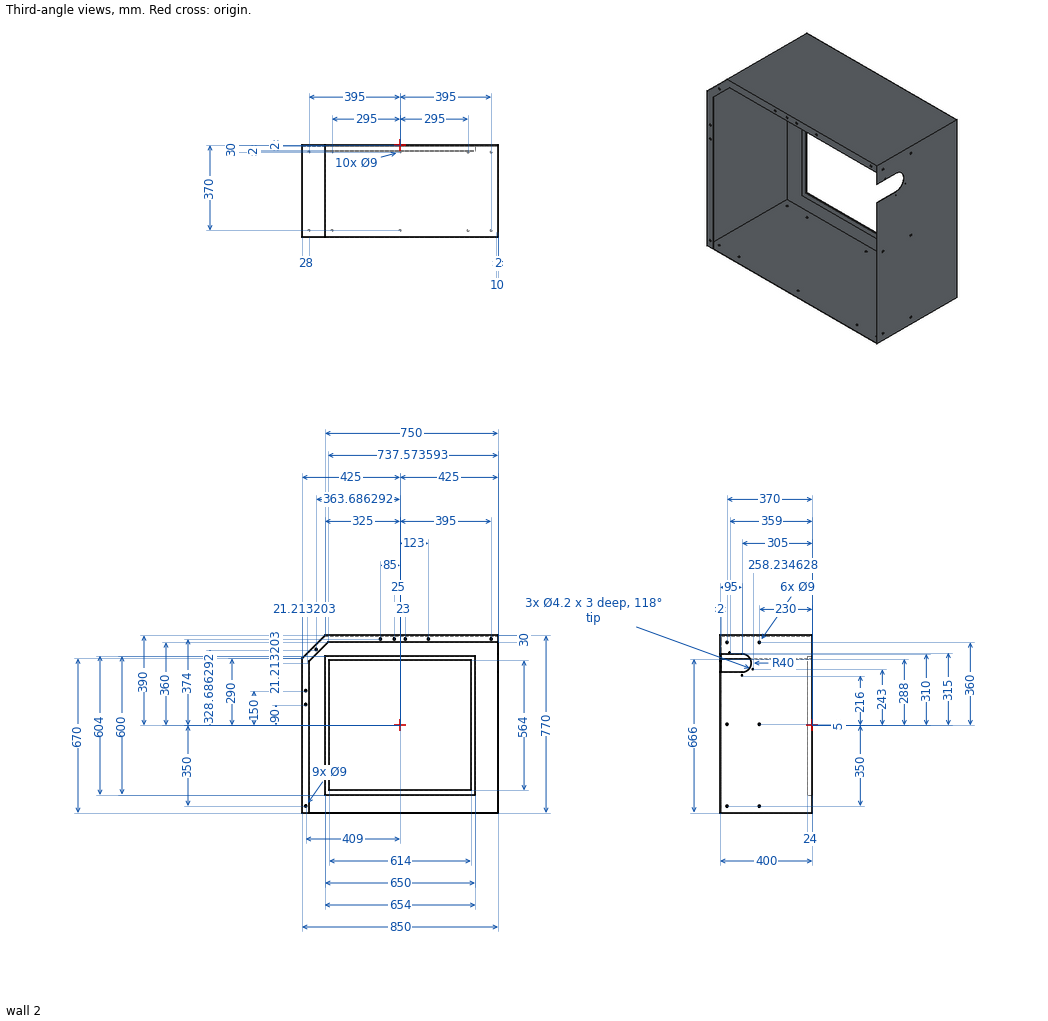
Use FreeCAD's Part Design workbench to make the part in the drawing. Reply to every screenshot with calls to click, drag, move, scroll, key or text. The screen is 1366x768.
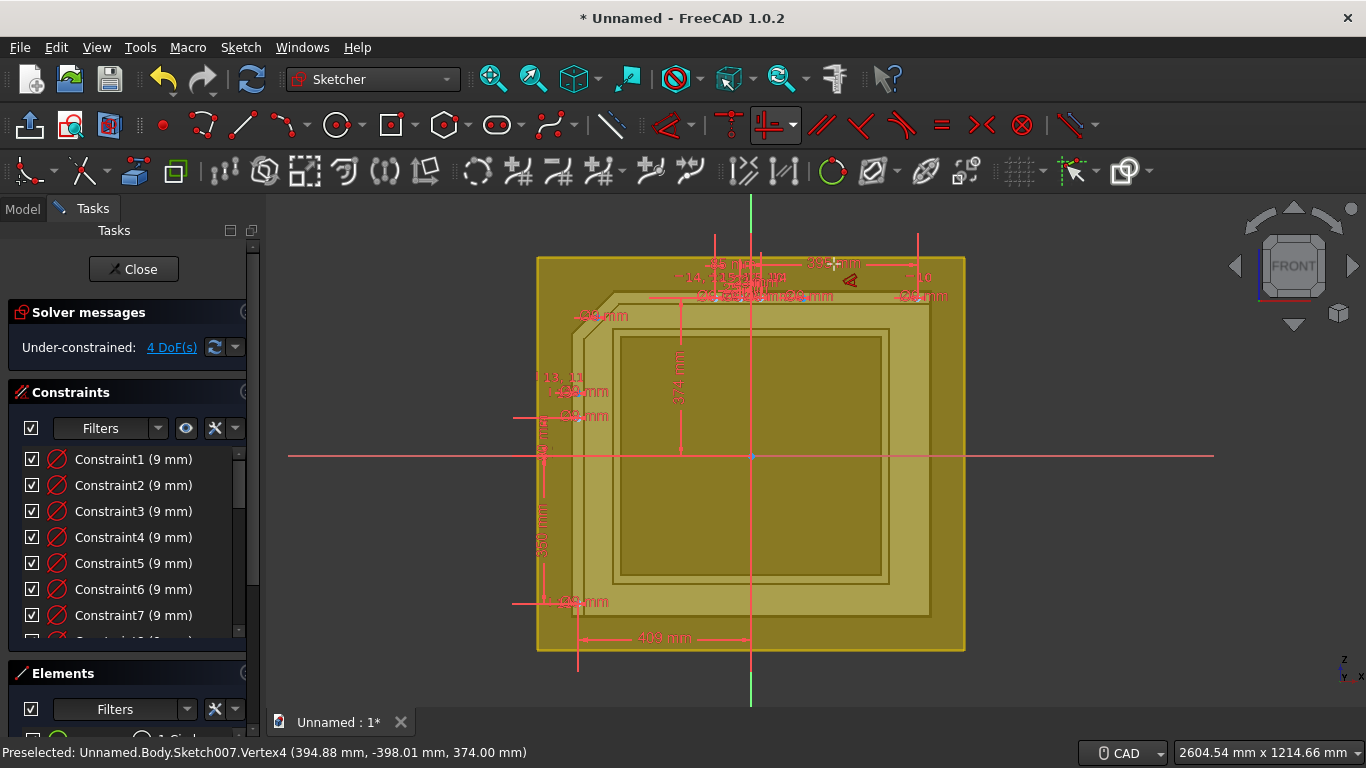
click(578, 393)
click(544, 410)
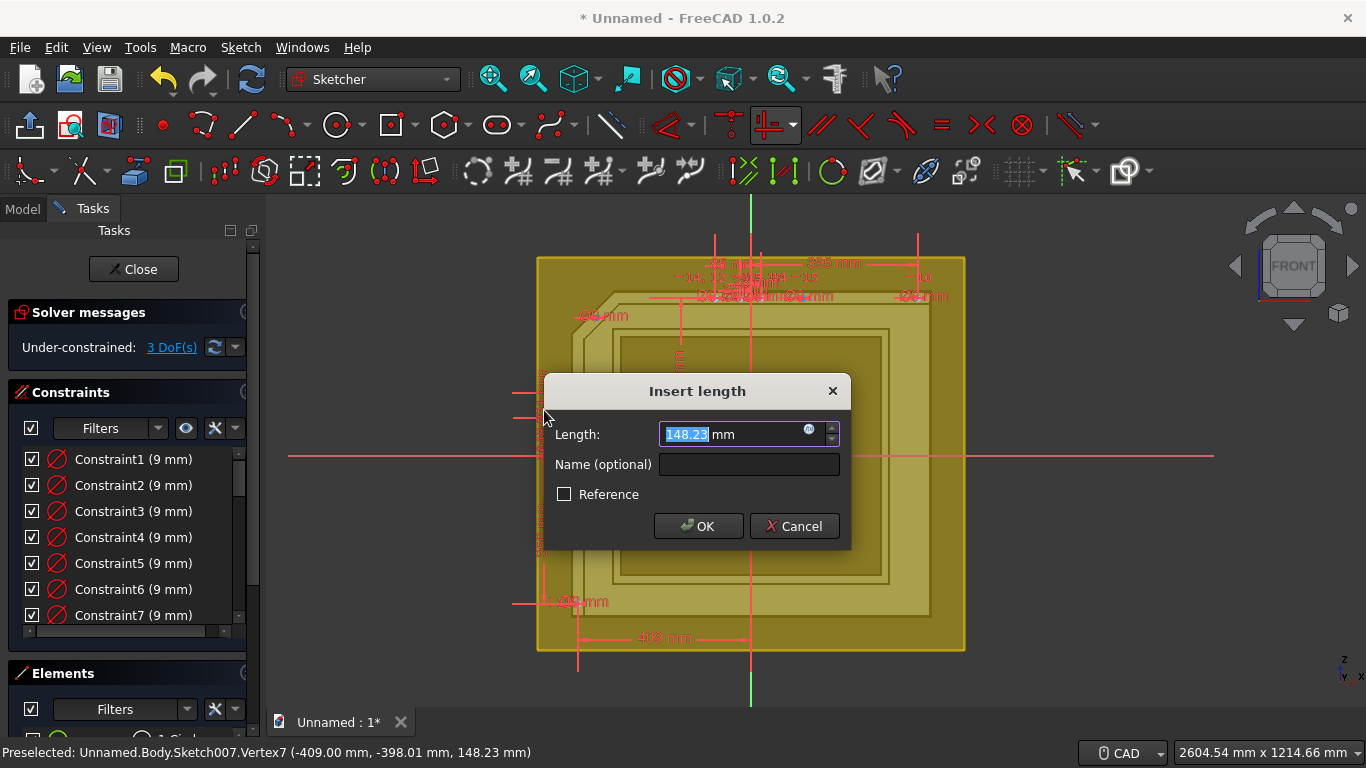
text(150)
key(Return)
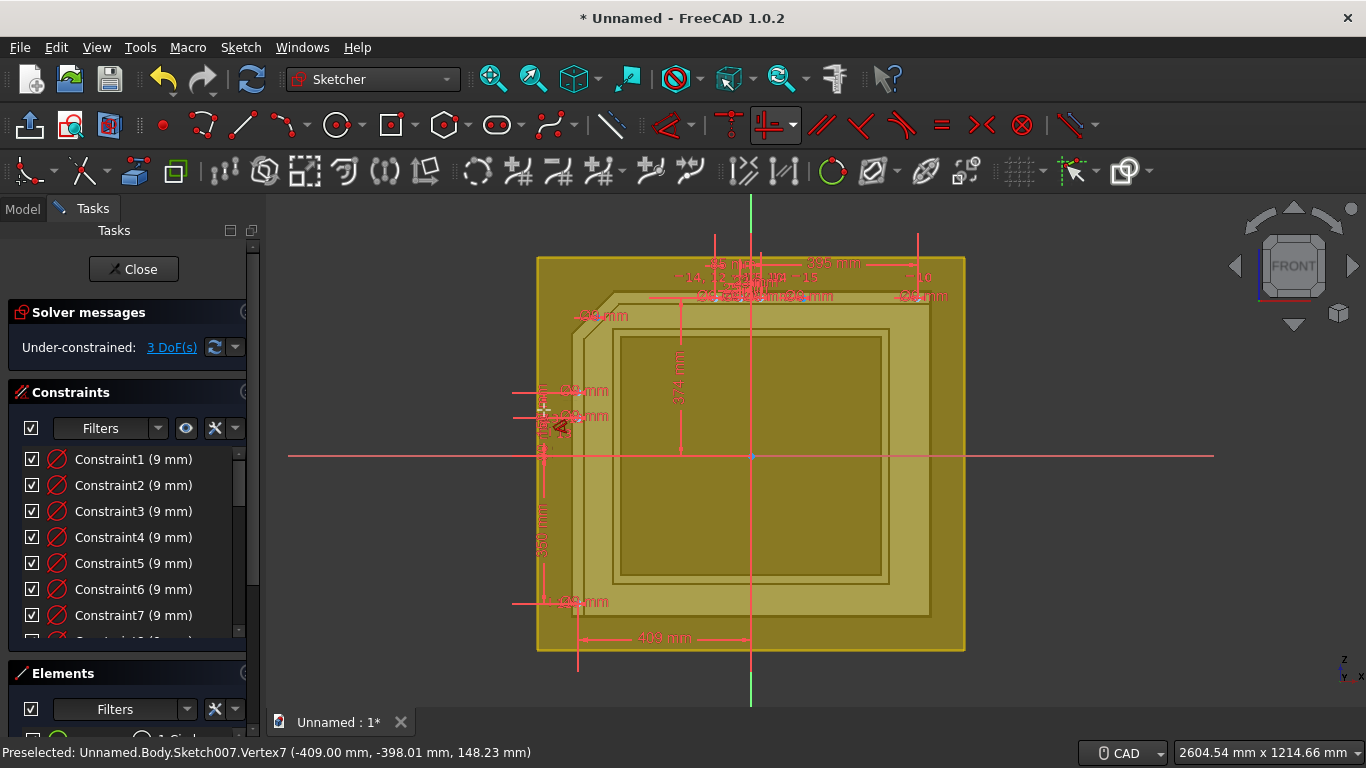
click(803, 298)
click(777, 490)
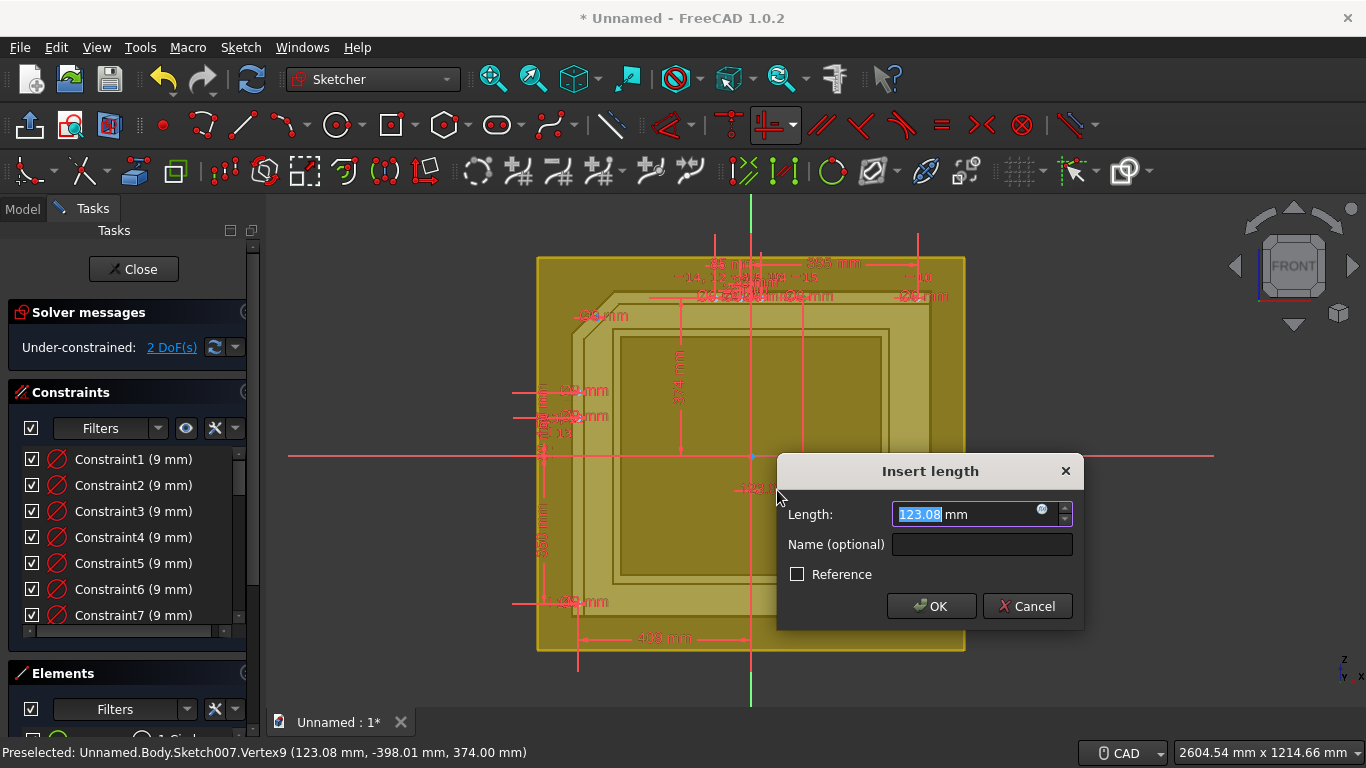
text(123)
key(Return)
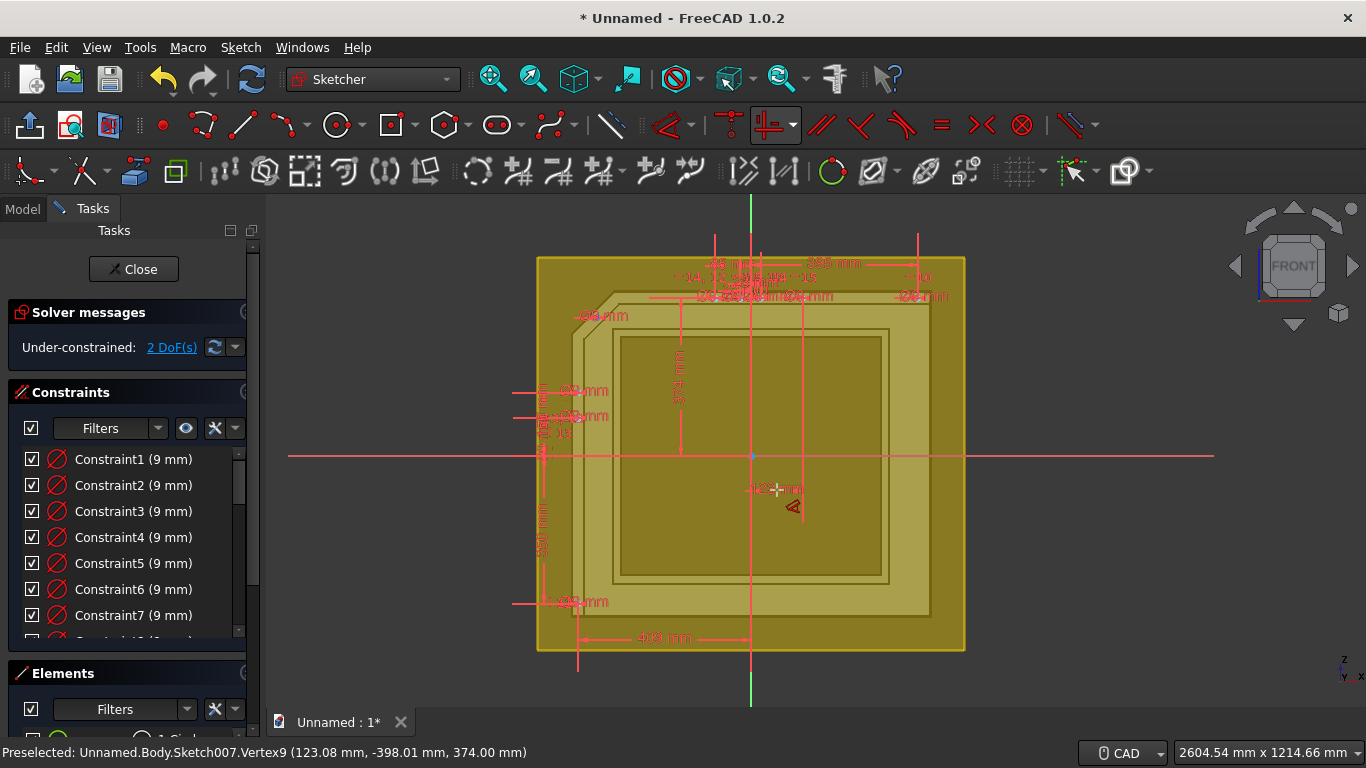
click(598, 318)
click(639, 284)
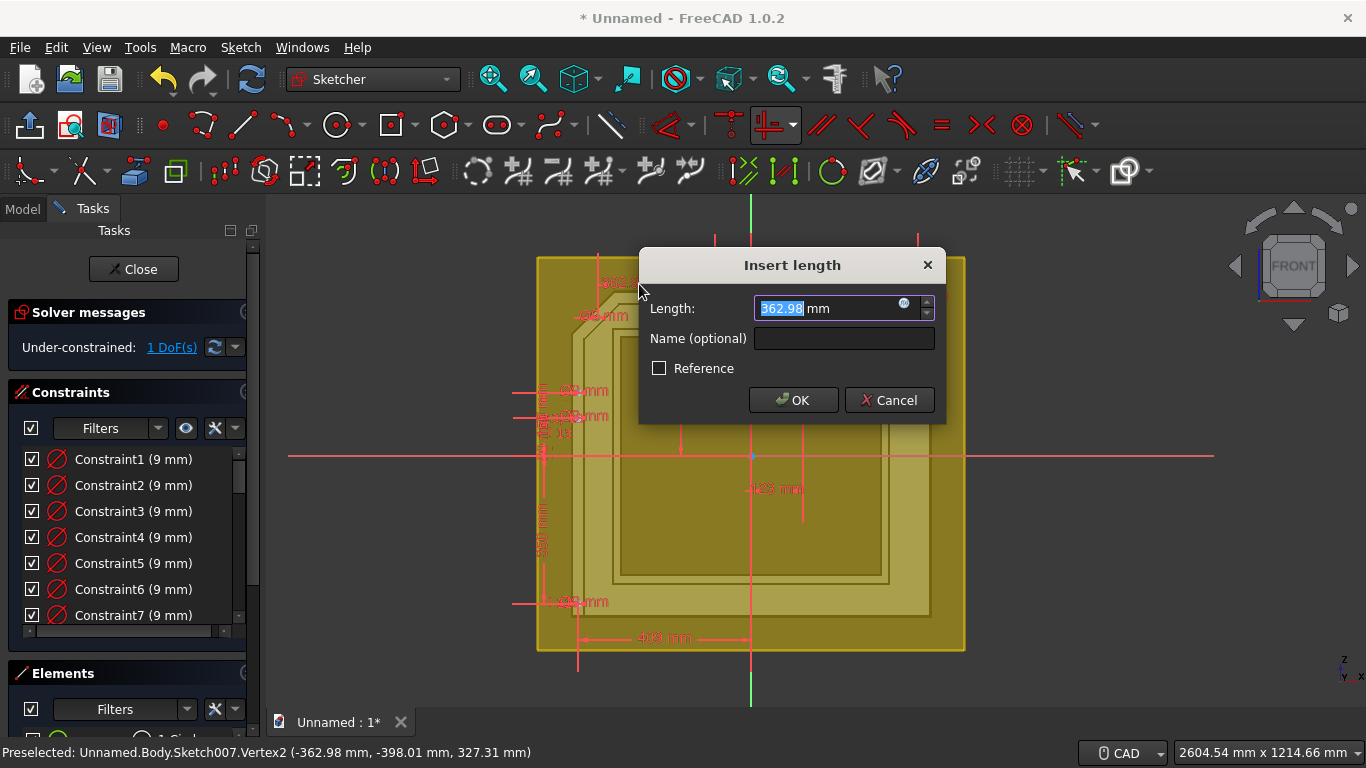
text(363.686292)
key(Return)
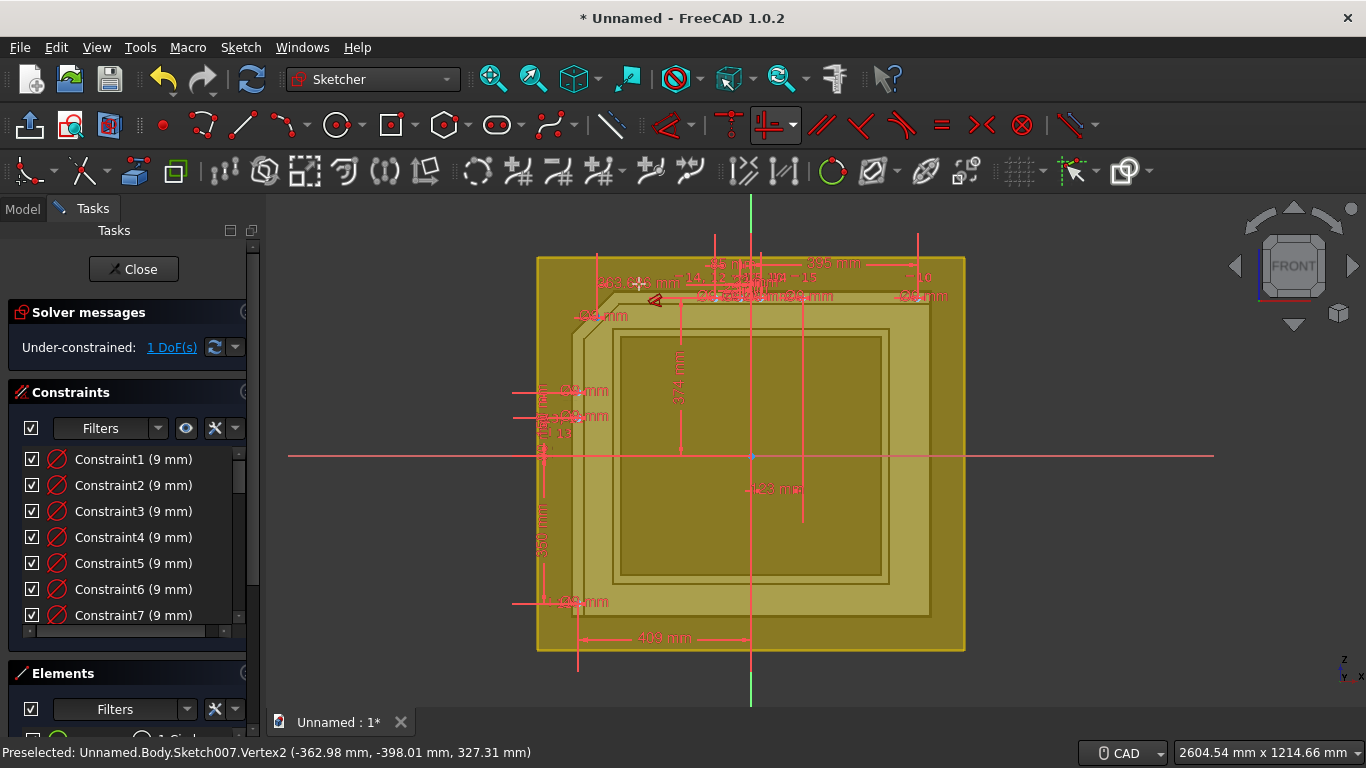
click(597, 318)
click(563, 387)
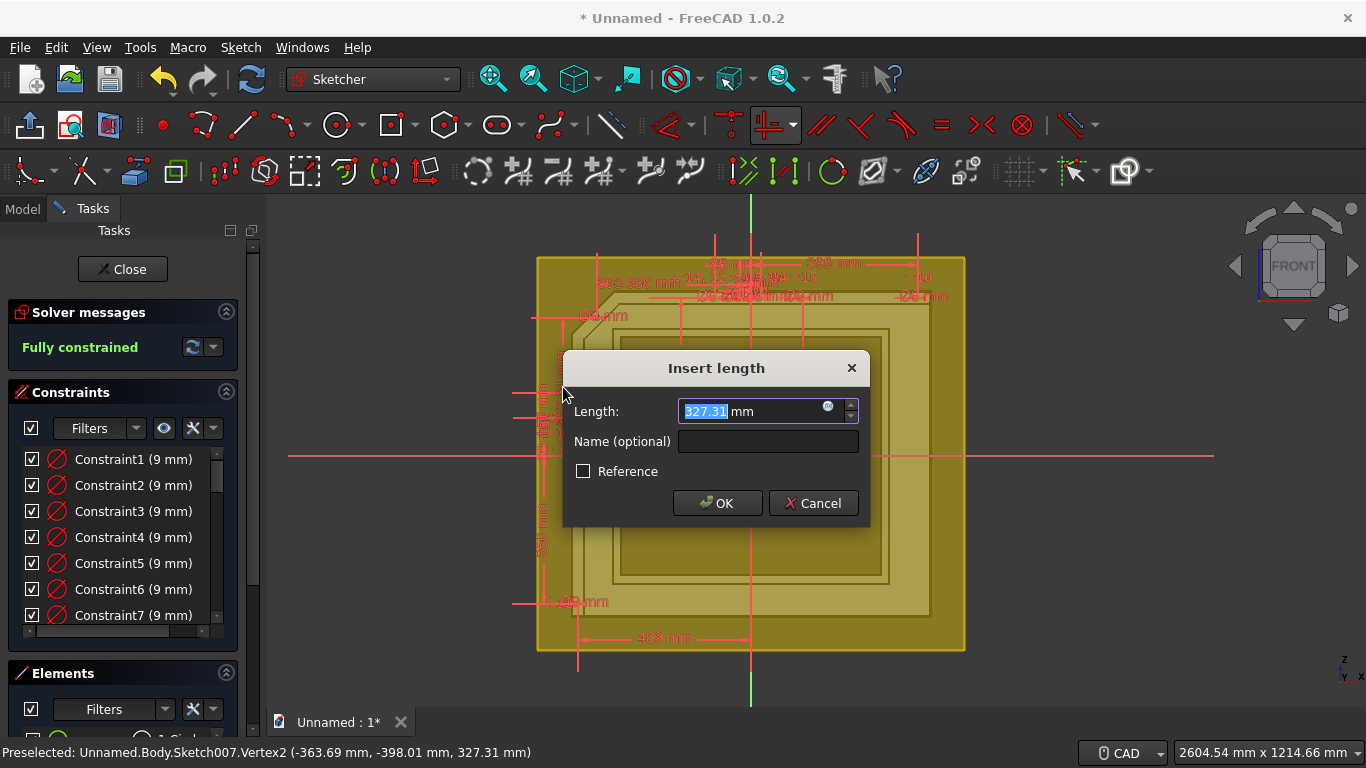
text(328.686292)
key(Return)
key(Escape)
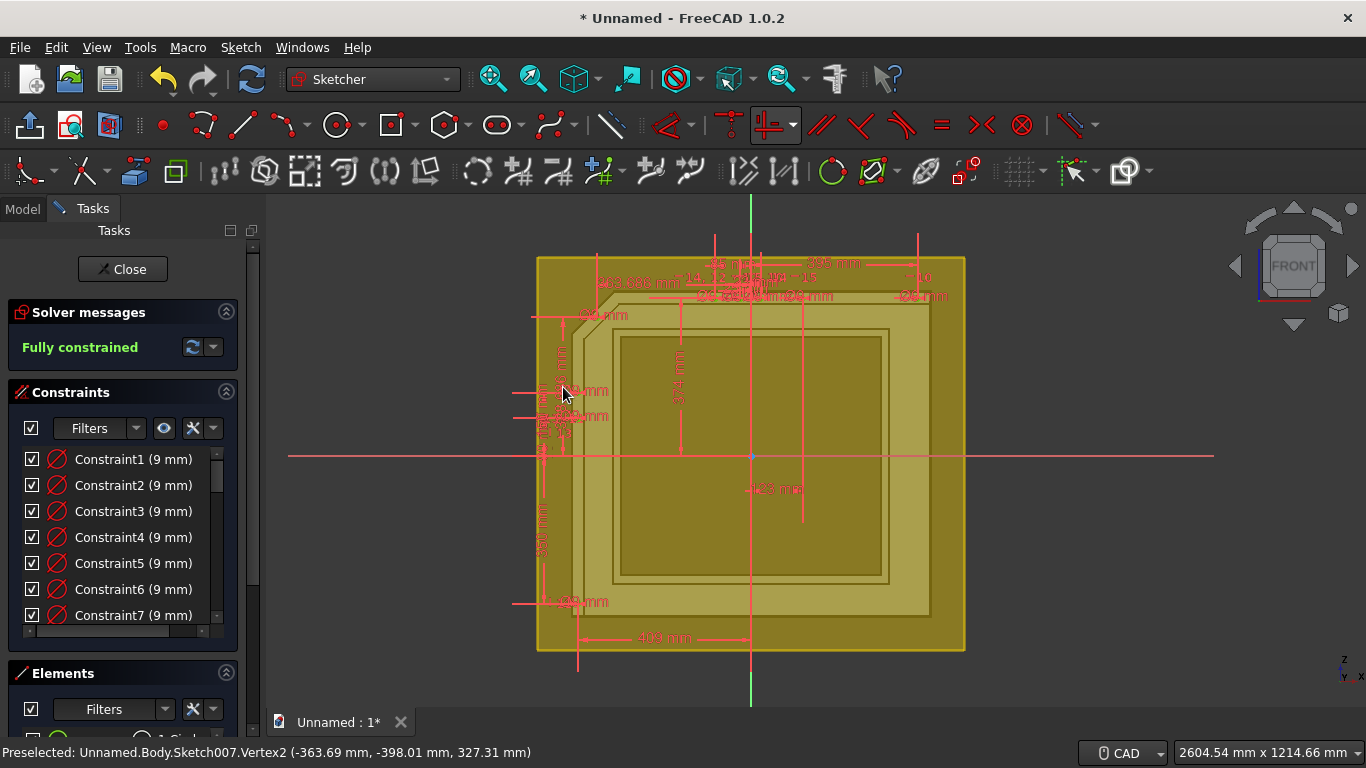
click(123, 269)